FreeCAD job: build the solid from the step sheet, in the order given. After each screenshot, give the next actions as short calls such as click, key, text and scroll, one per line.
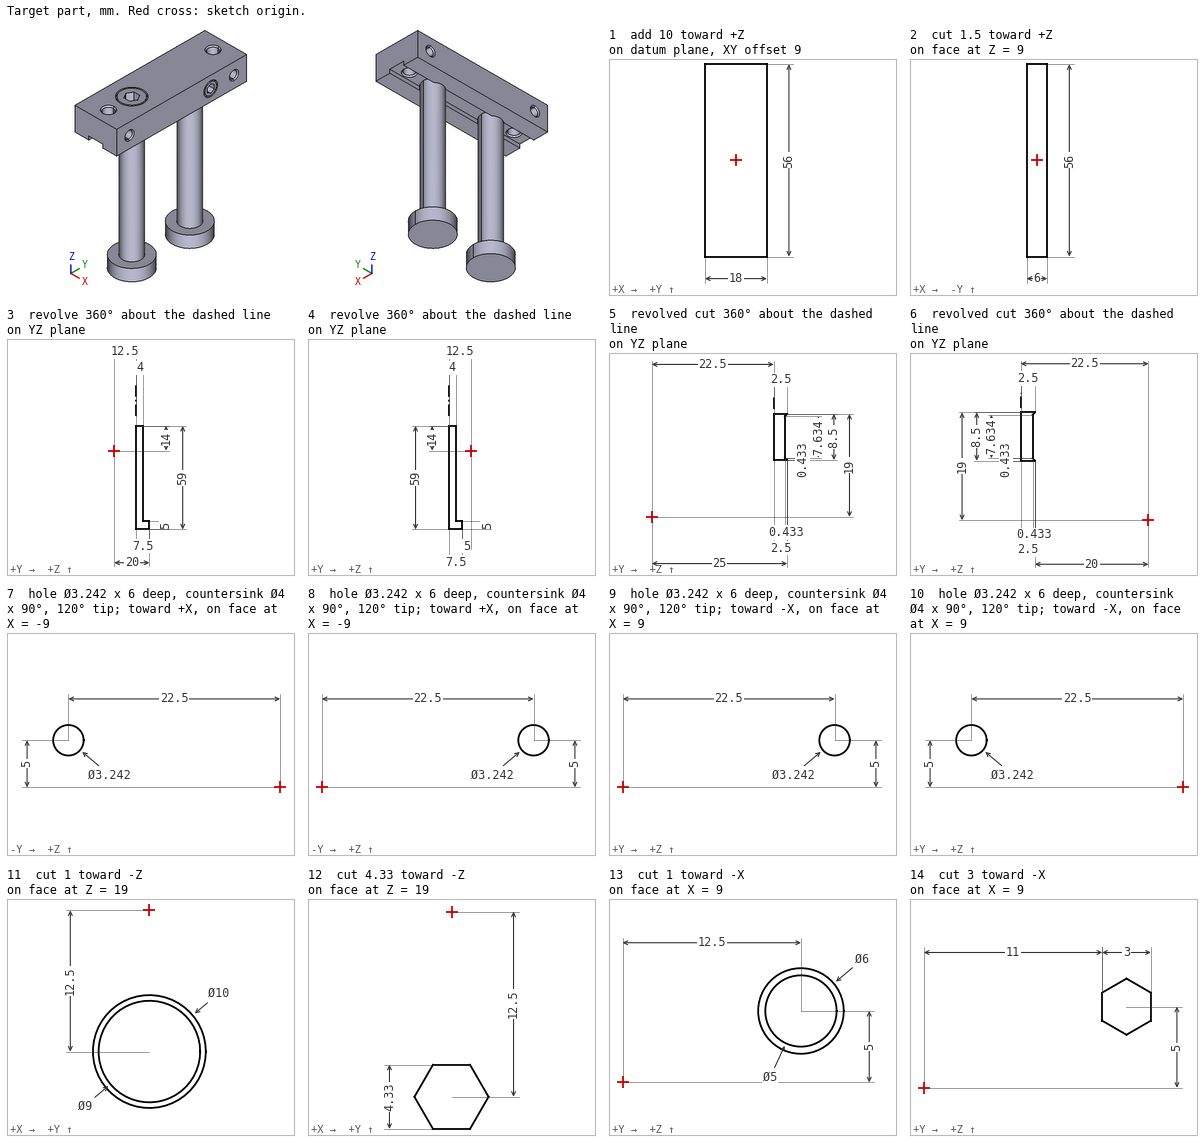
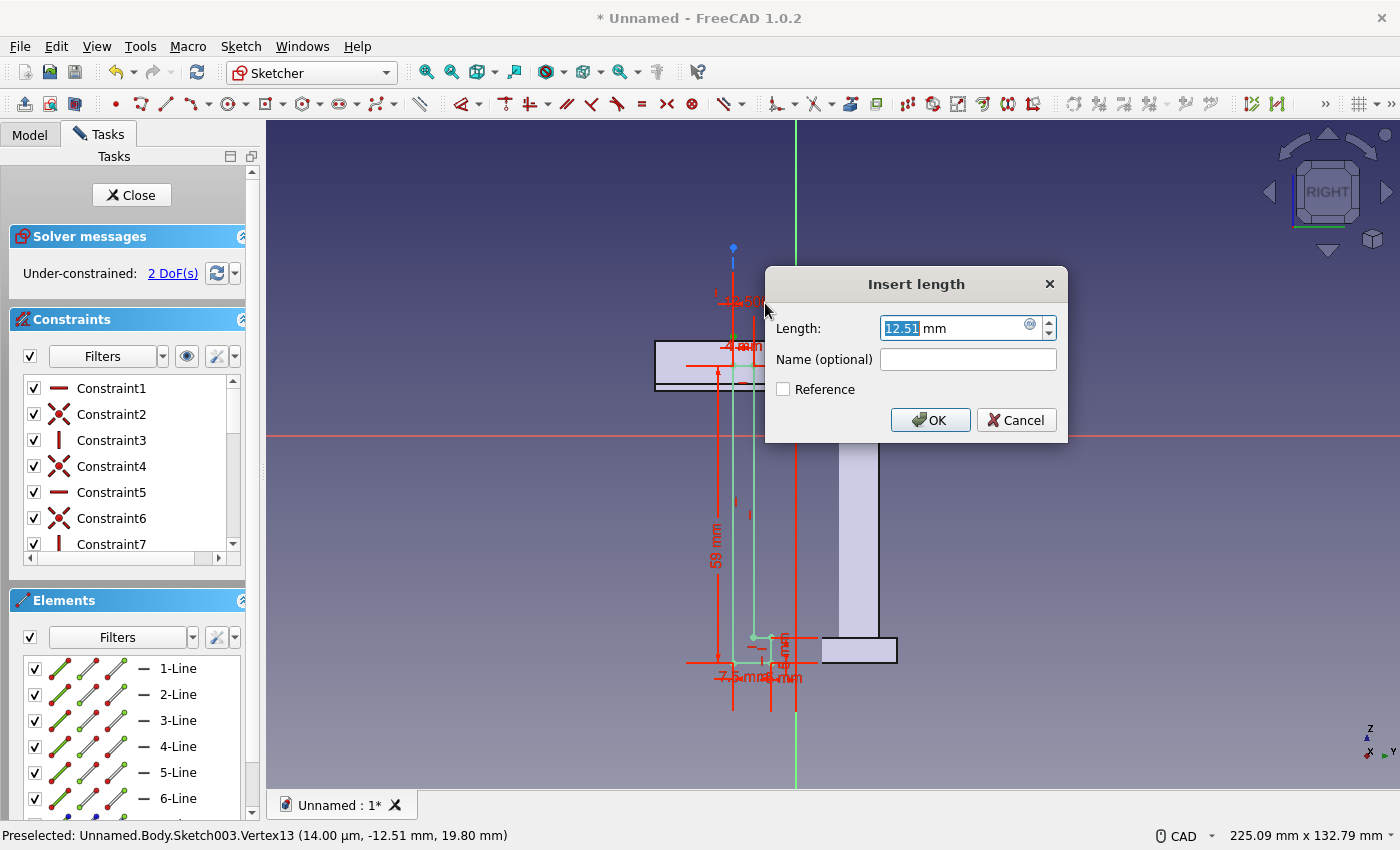
text(12.5)
key(Return)
key(Escape)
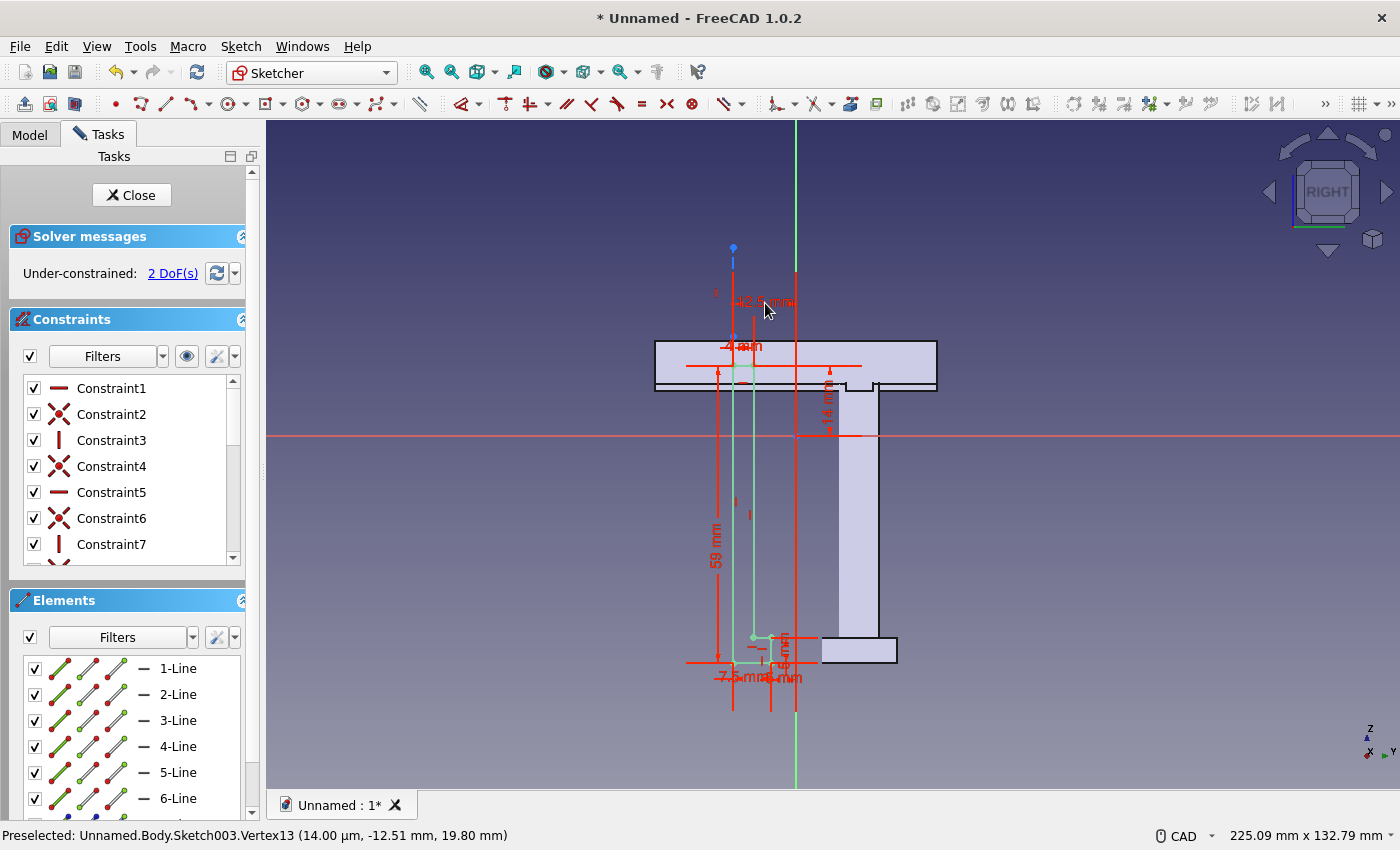
click(132, 195)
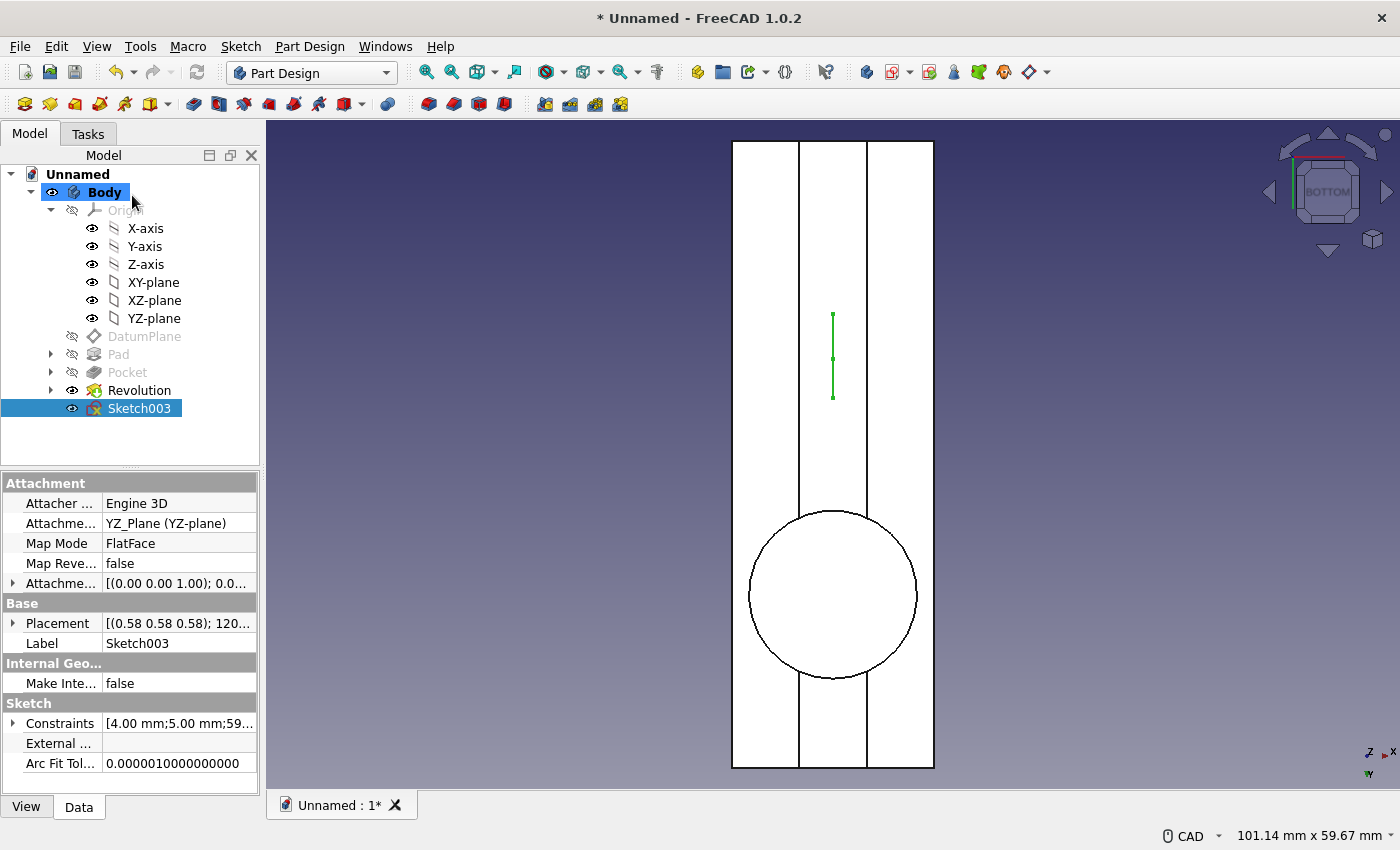
click(50, 104)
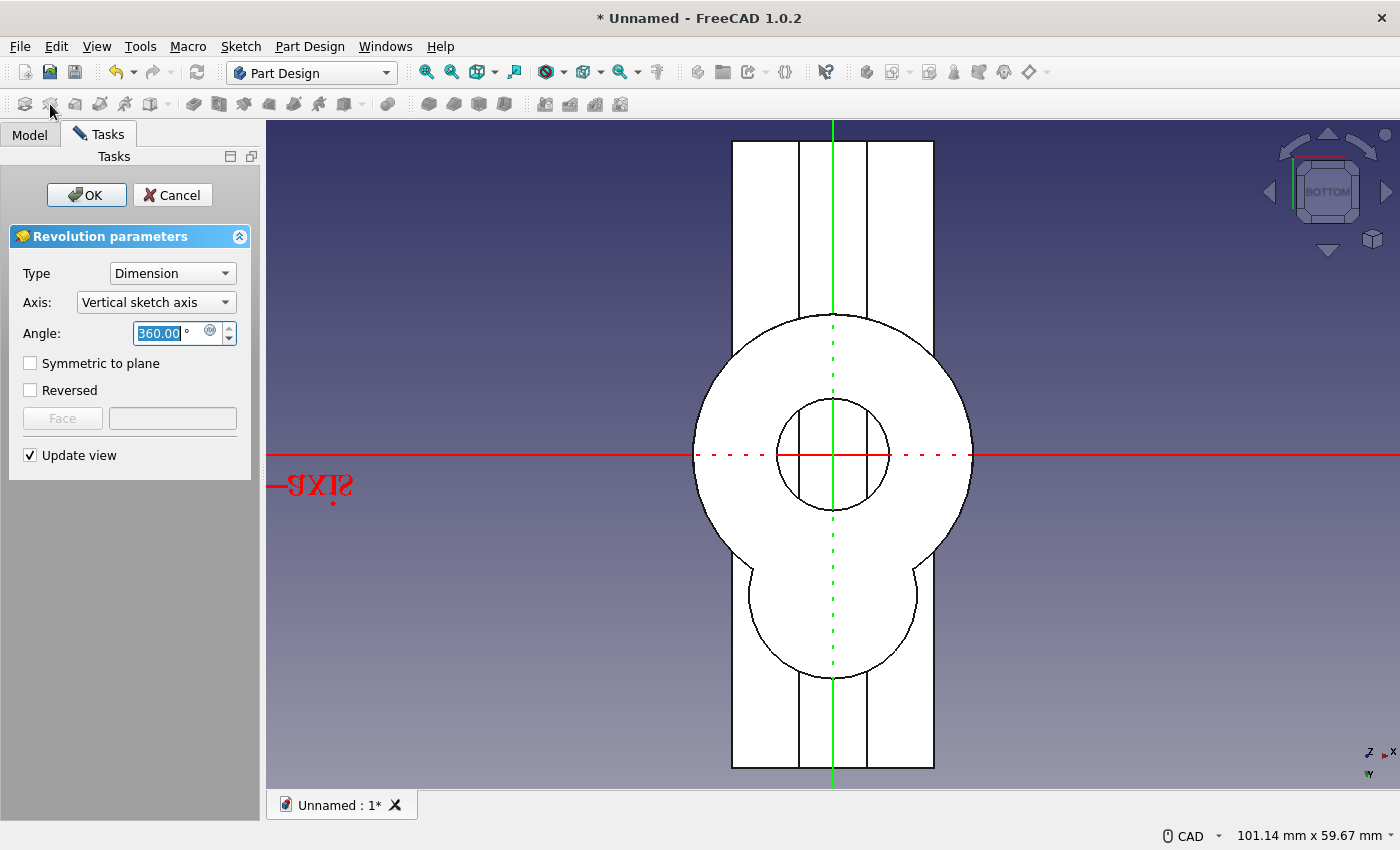
click(157, 302)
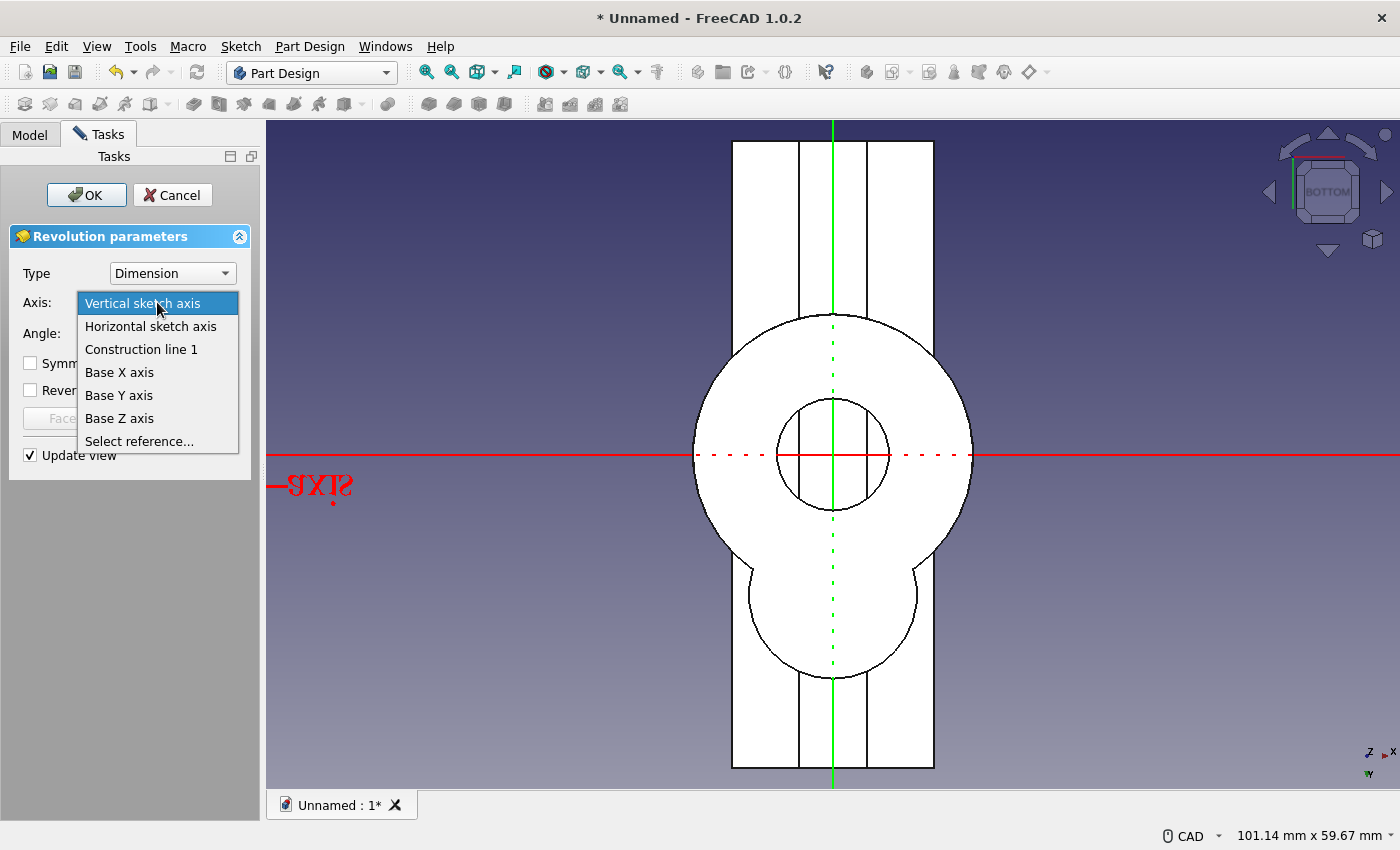
click(156, 350)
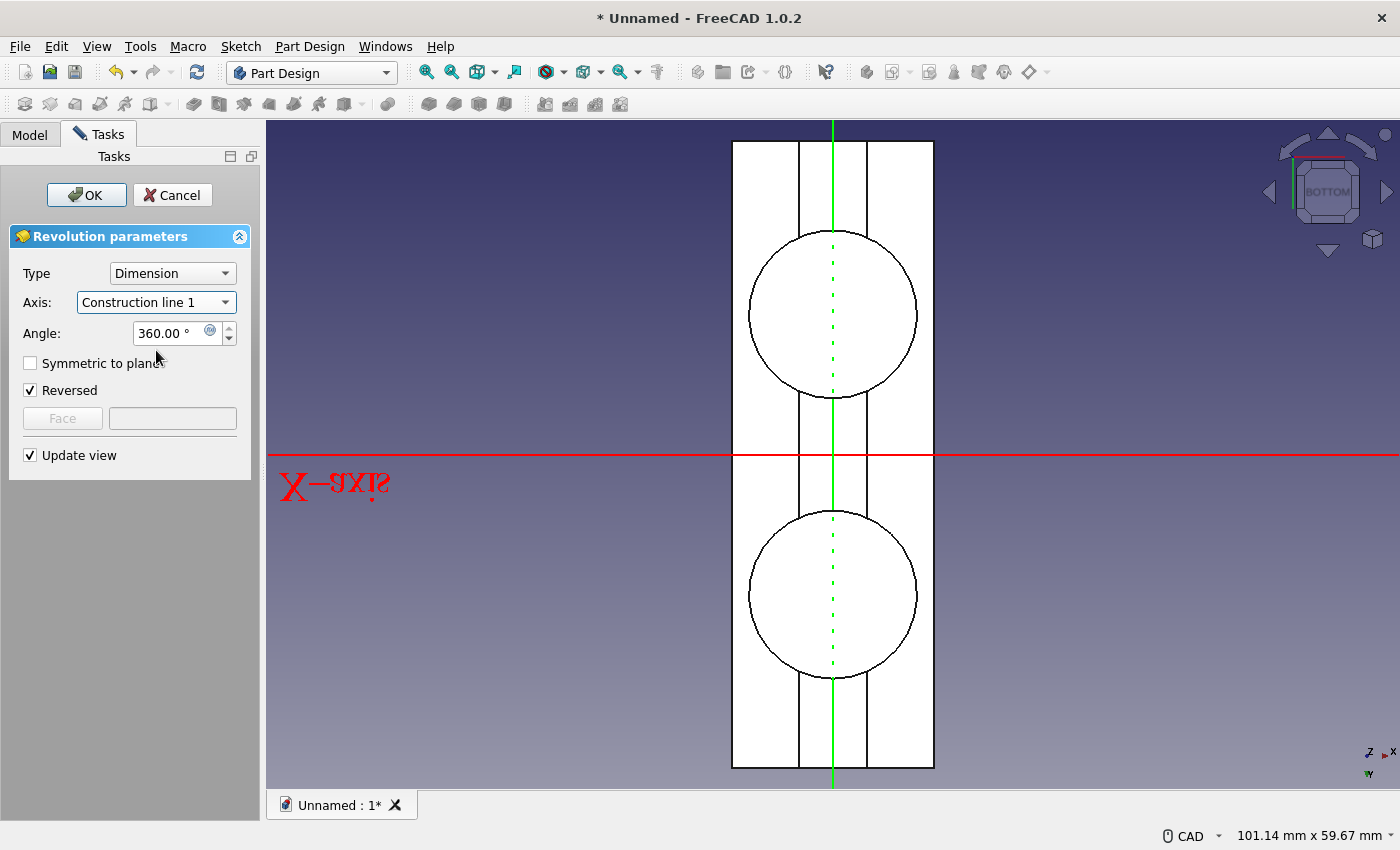
click(87, 195)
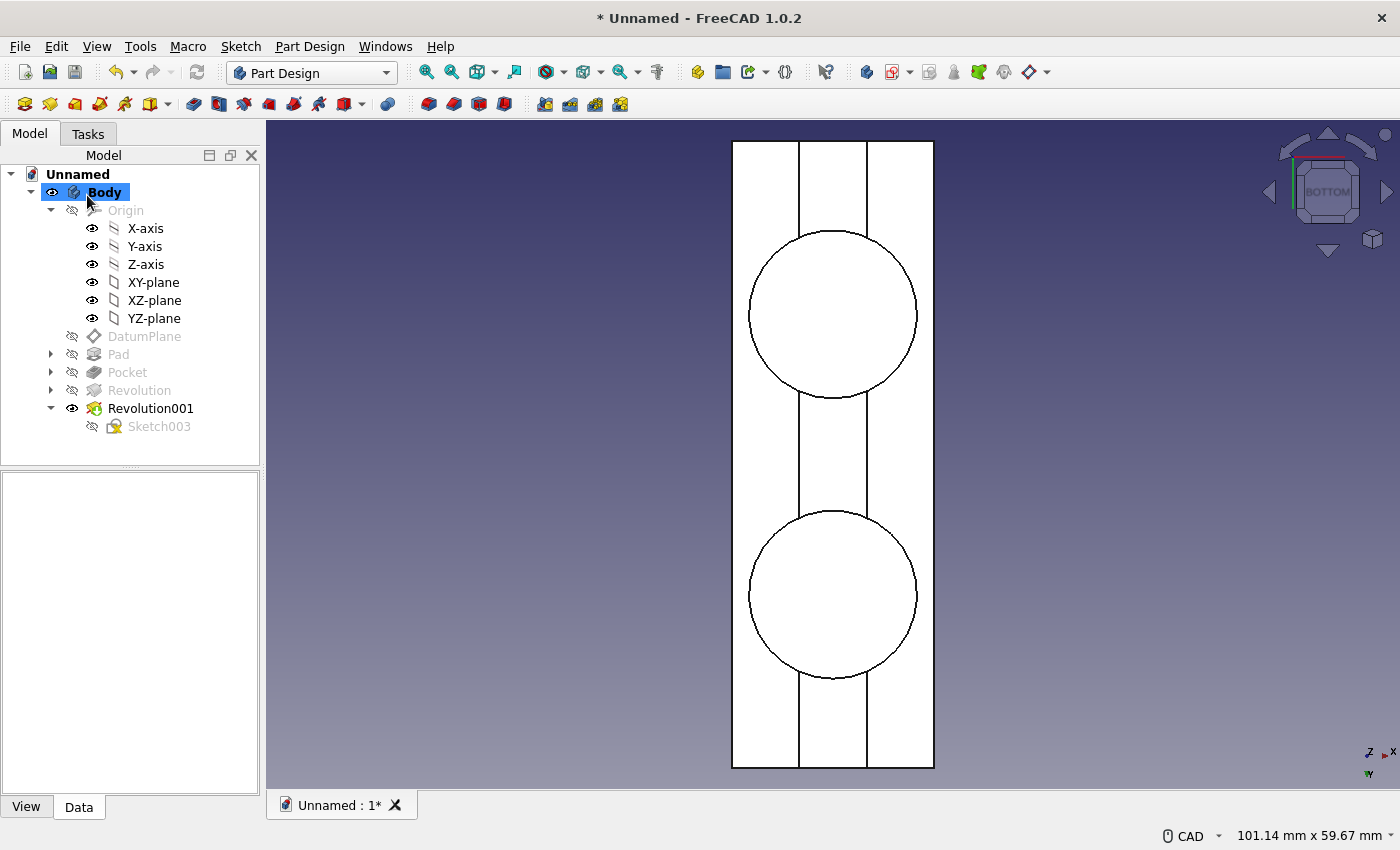
click(892, 72)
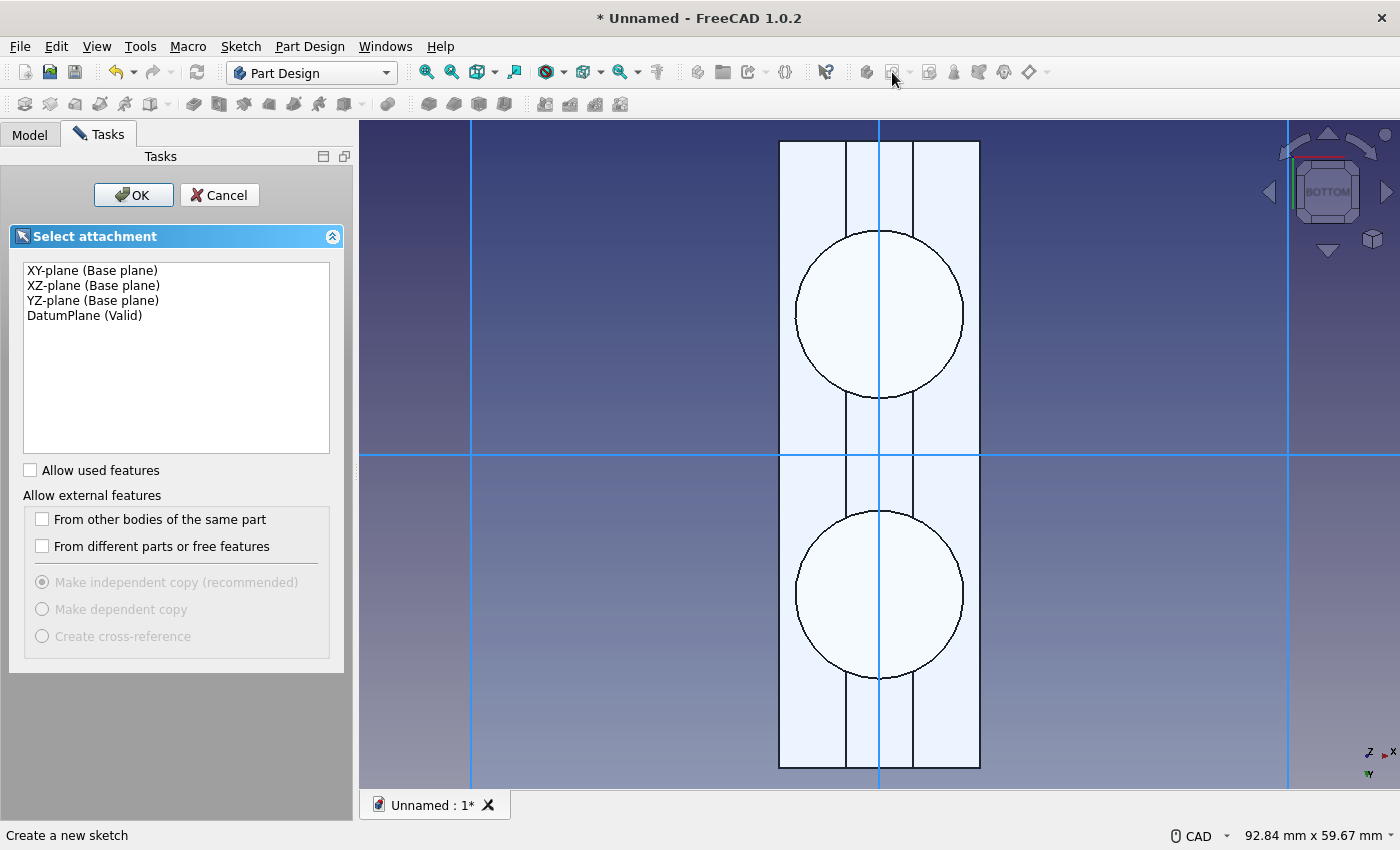
click(84, 300)